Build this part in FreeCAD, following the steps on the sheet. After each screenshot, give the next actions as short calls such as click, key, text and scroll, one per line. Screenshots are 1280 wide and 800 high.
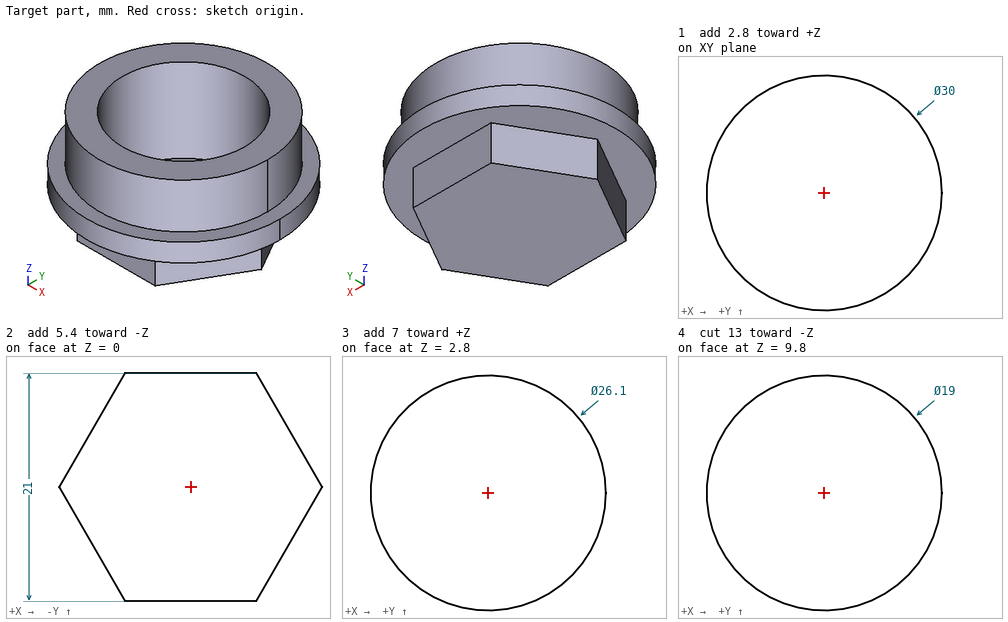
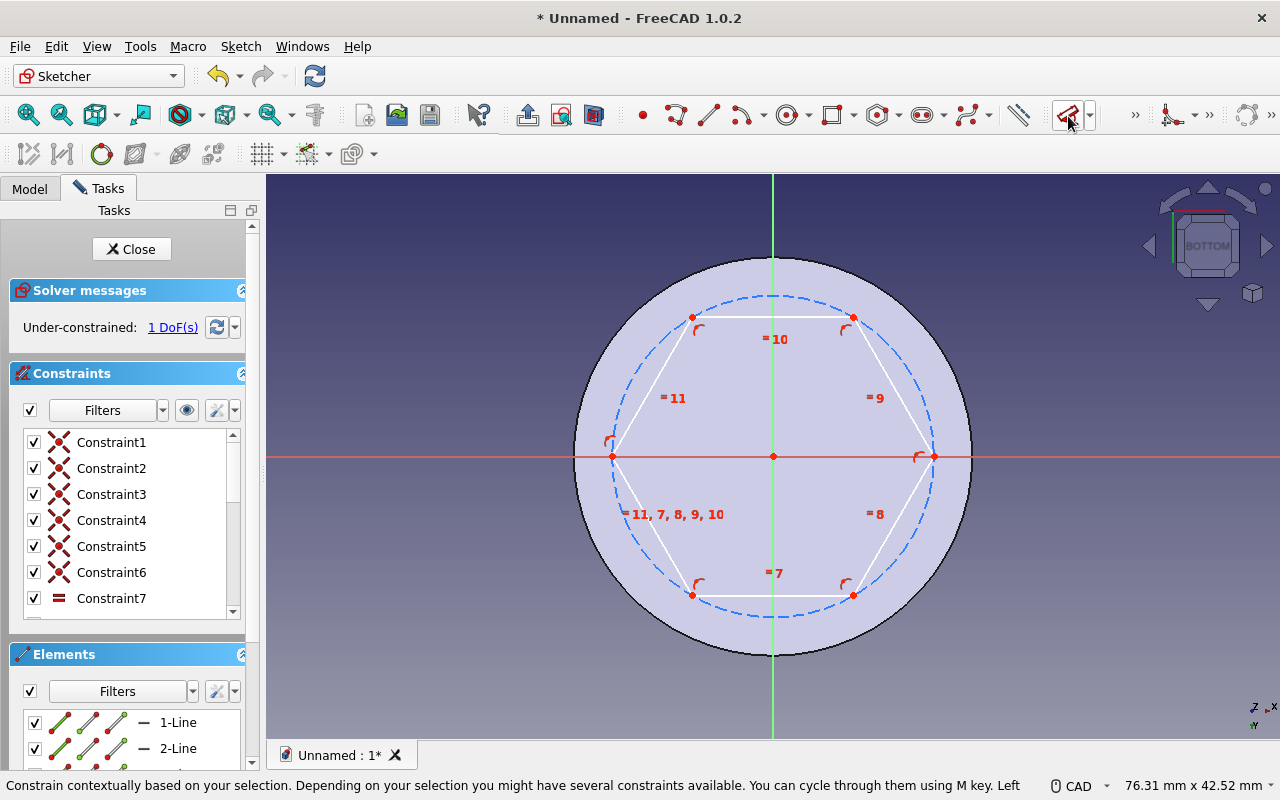
click(693, 596)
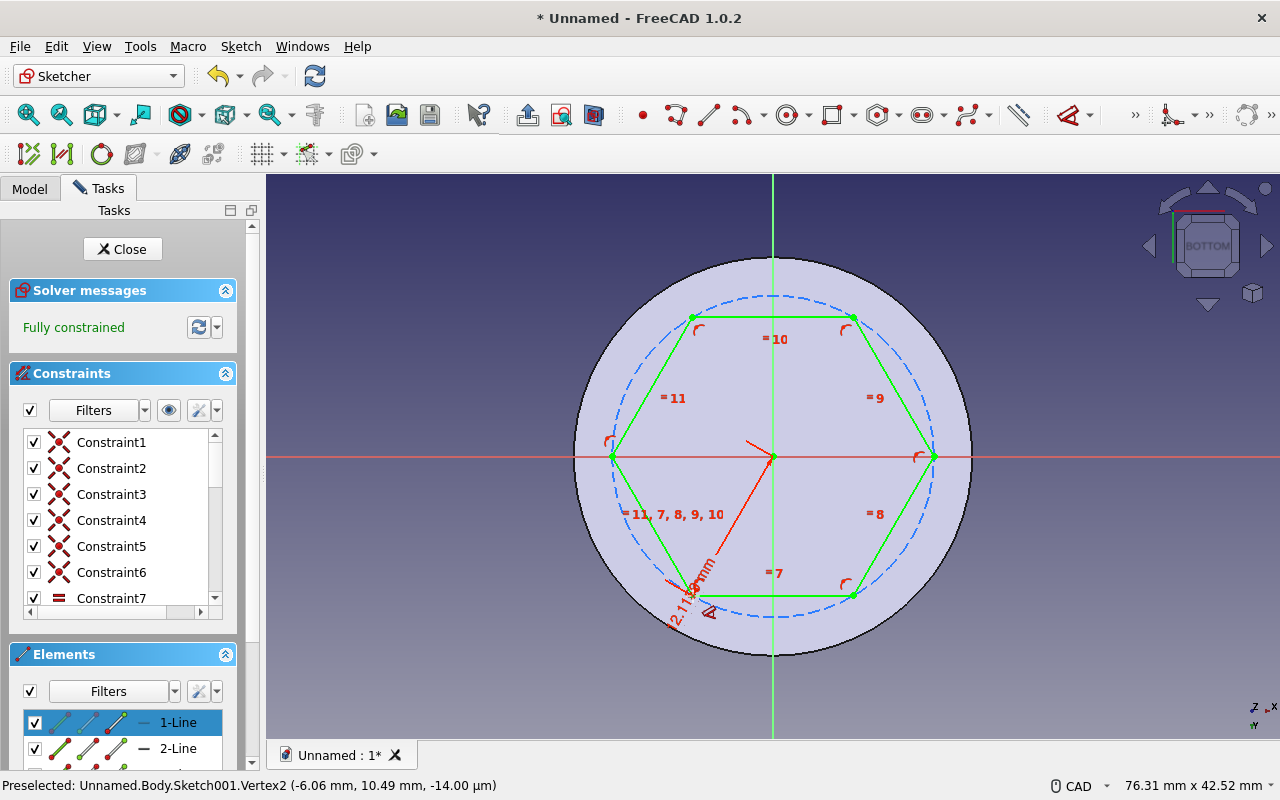
click(853, 317)
click(935, 392)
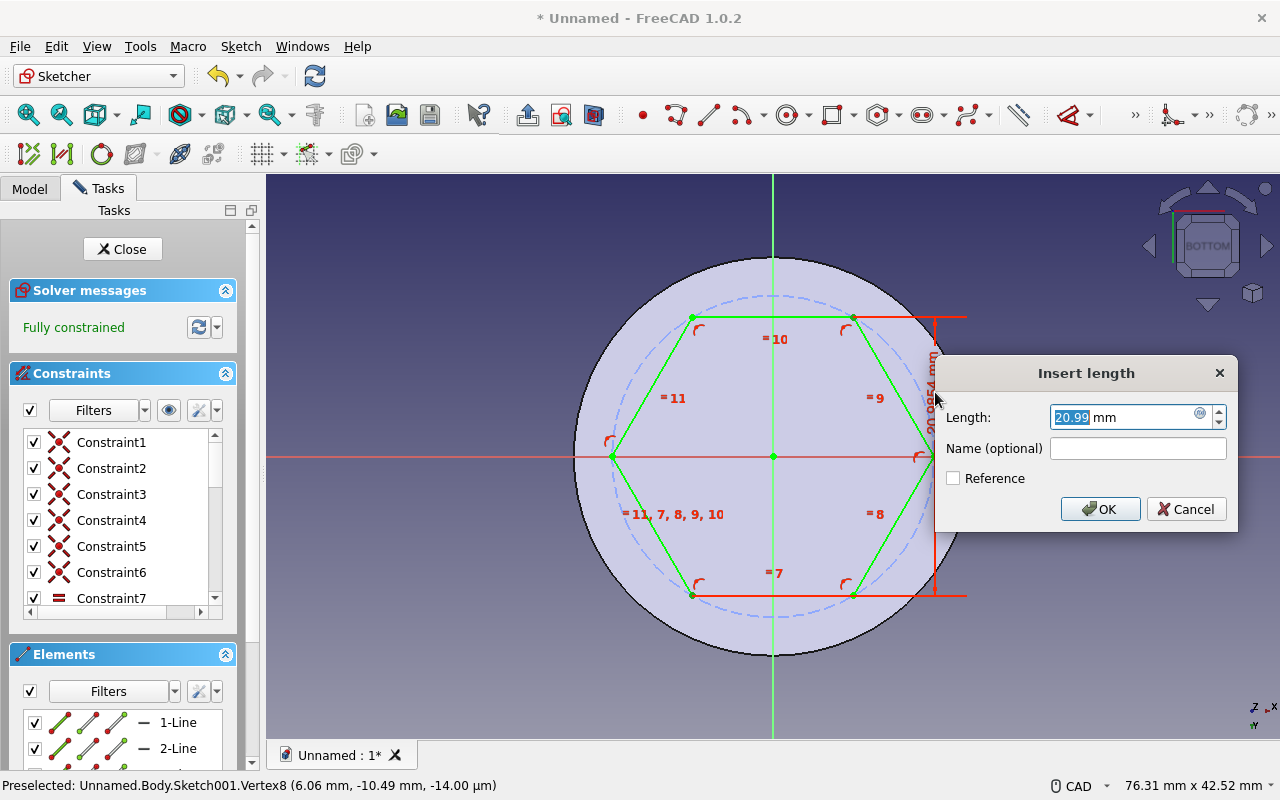
text(21)
key(Return)
key(Escape)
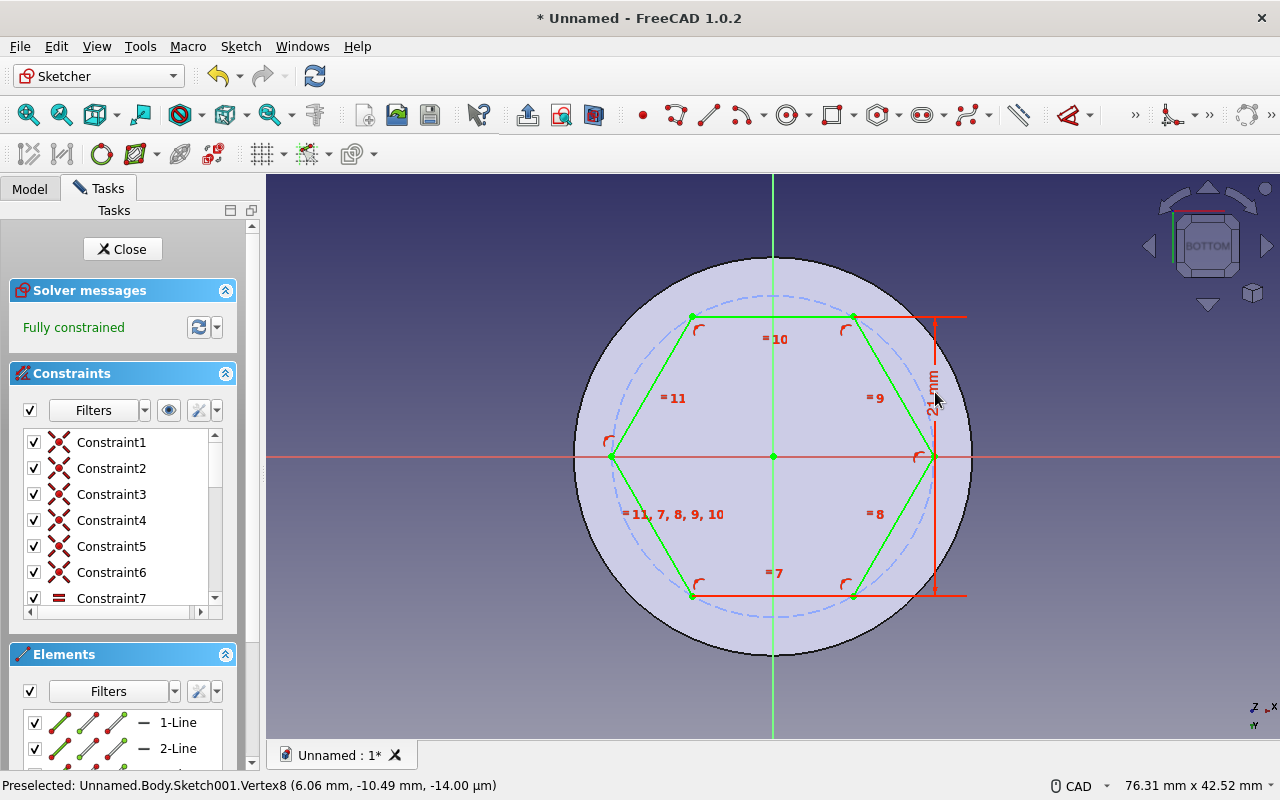
click(123, 249)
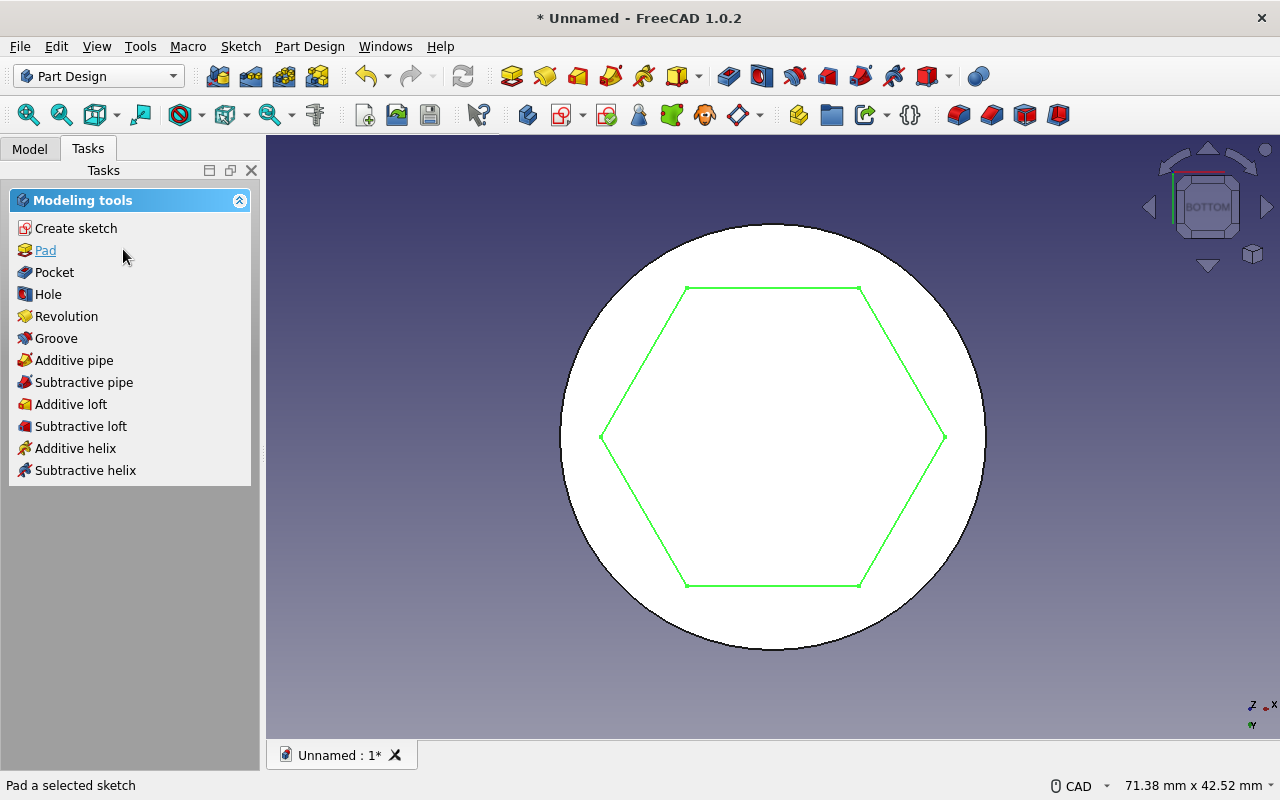
click(512, 76)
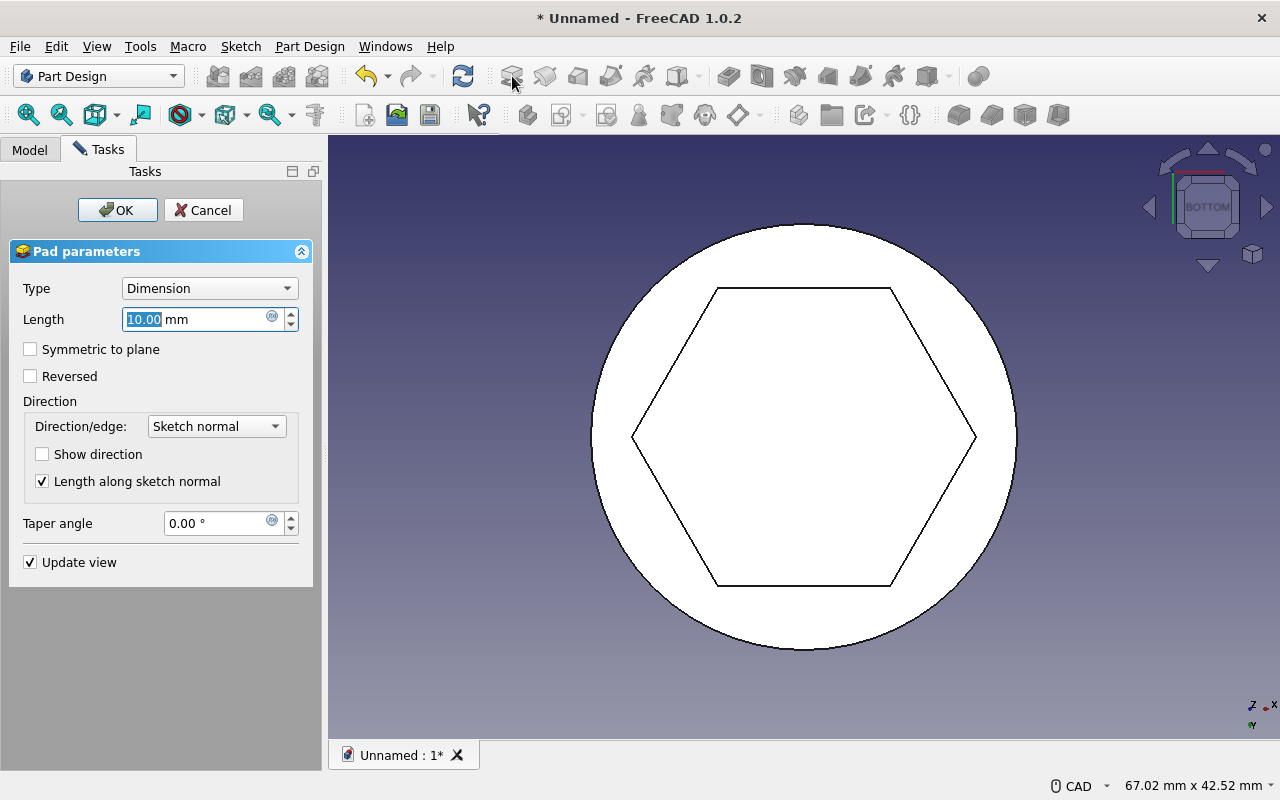
text(5.4)
key(Tab)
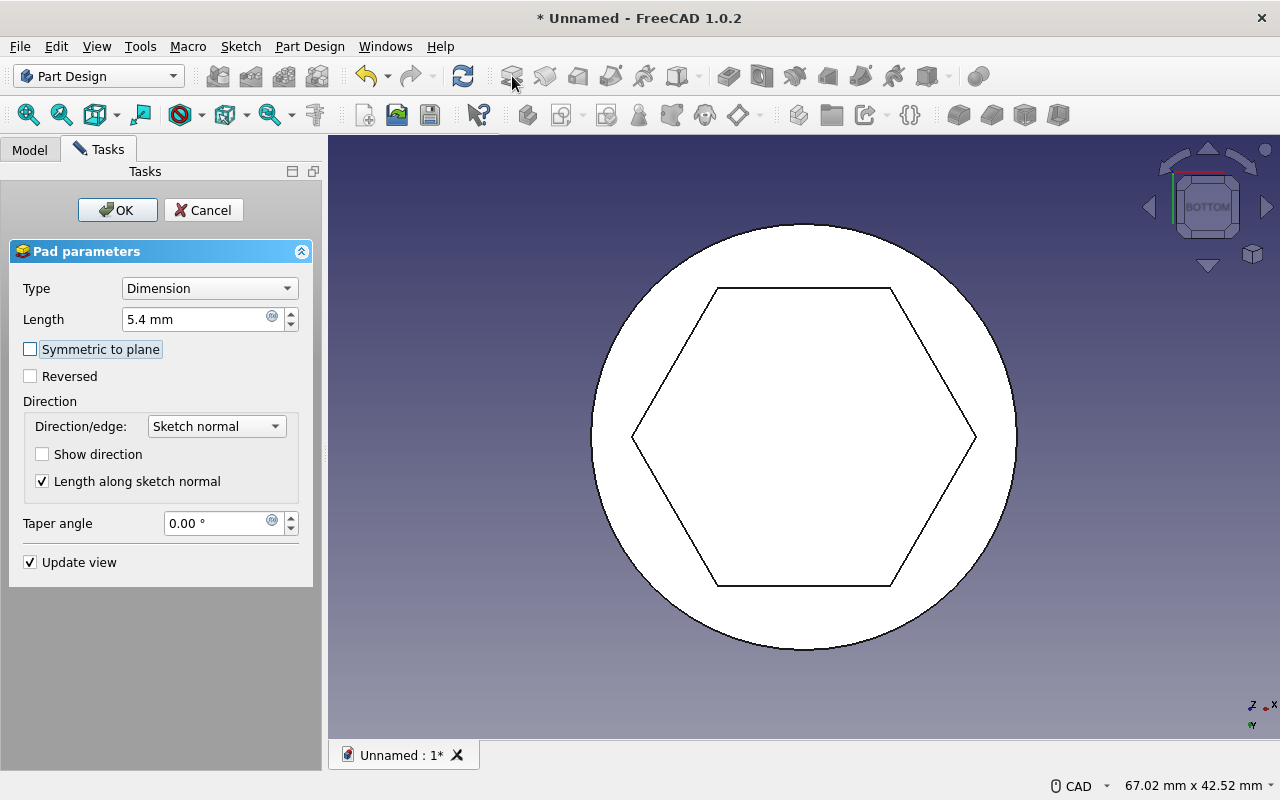
click(118, 210)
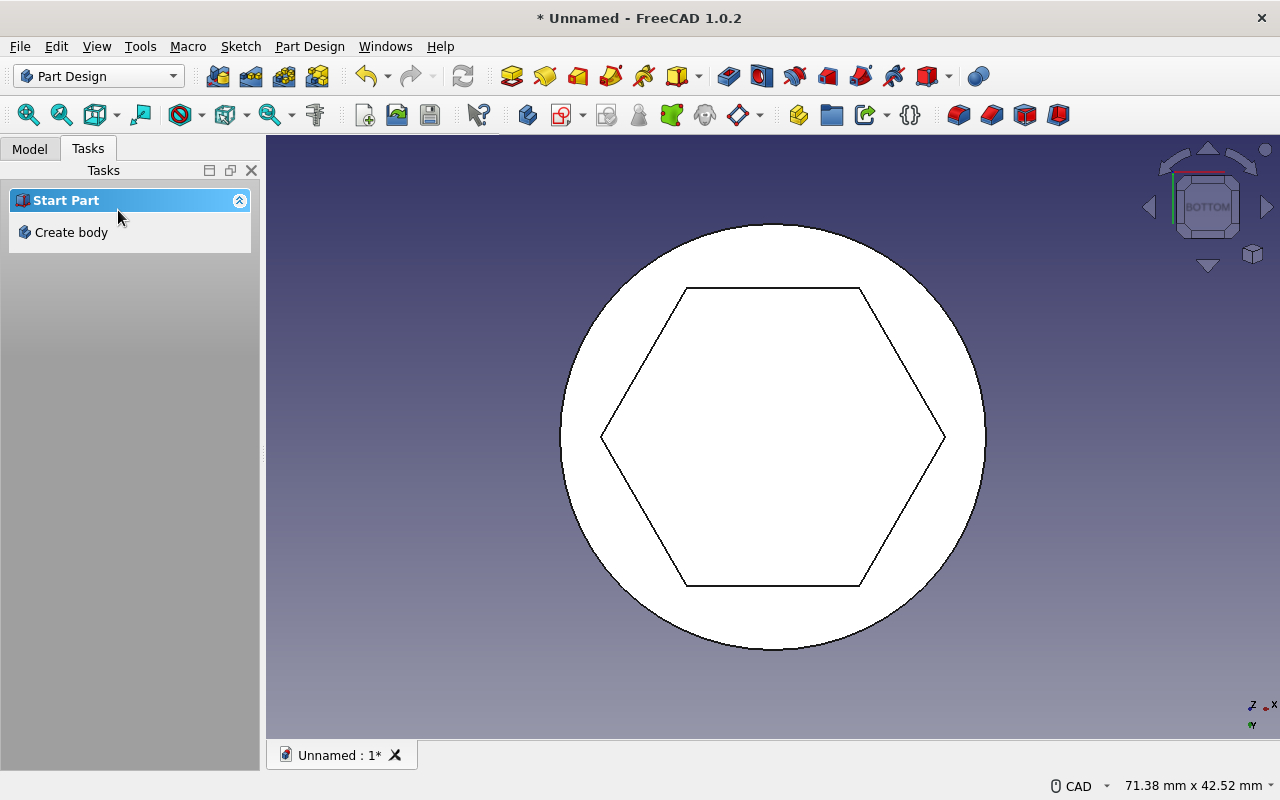
key(0)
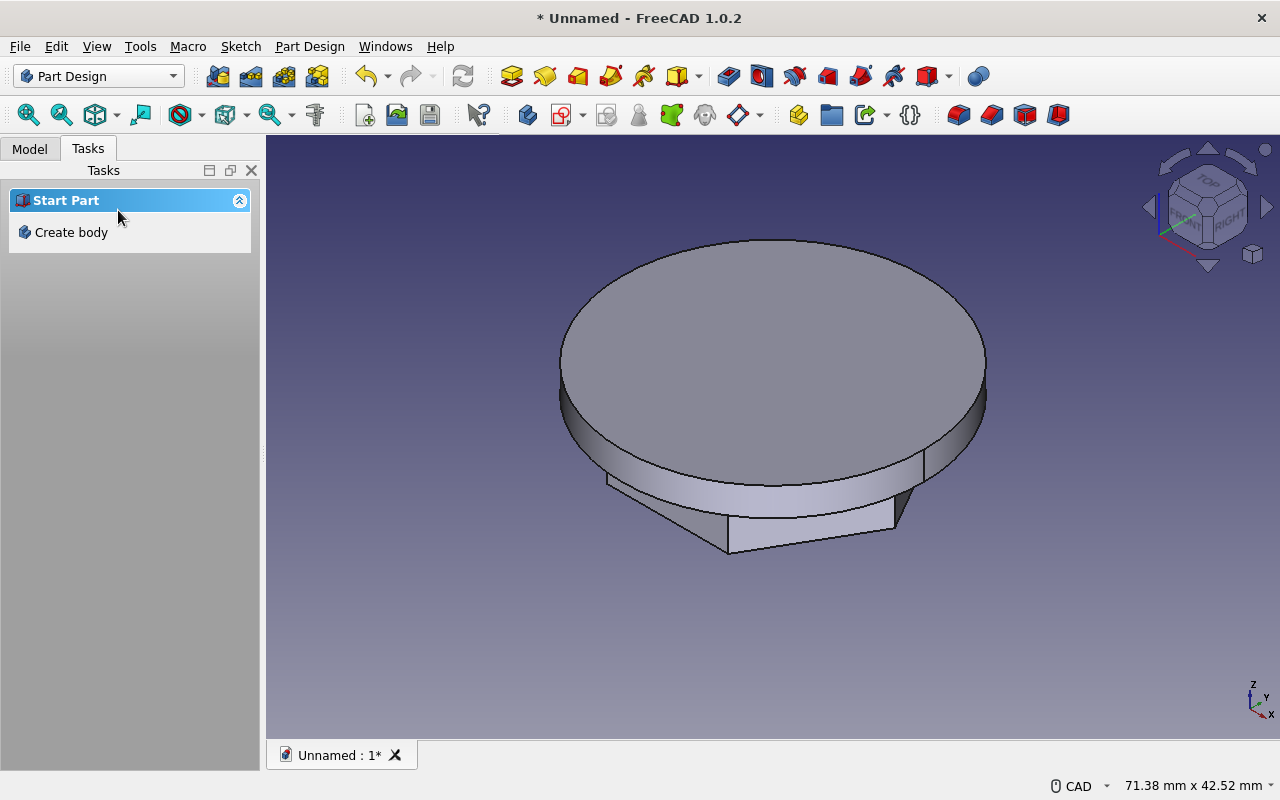
click(773, 362)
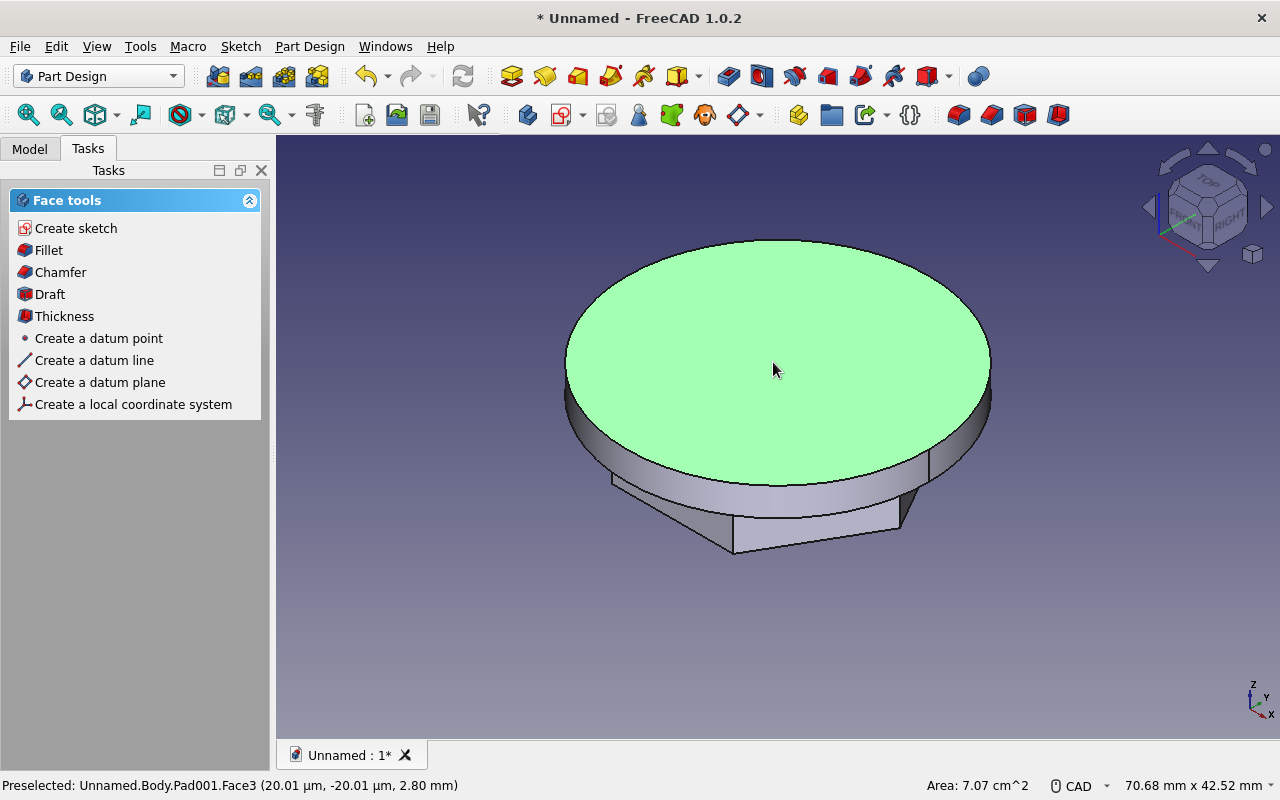
click(560, 116)